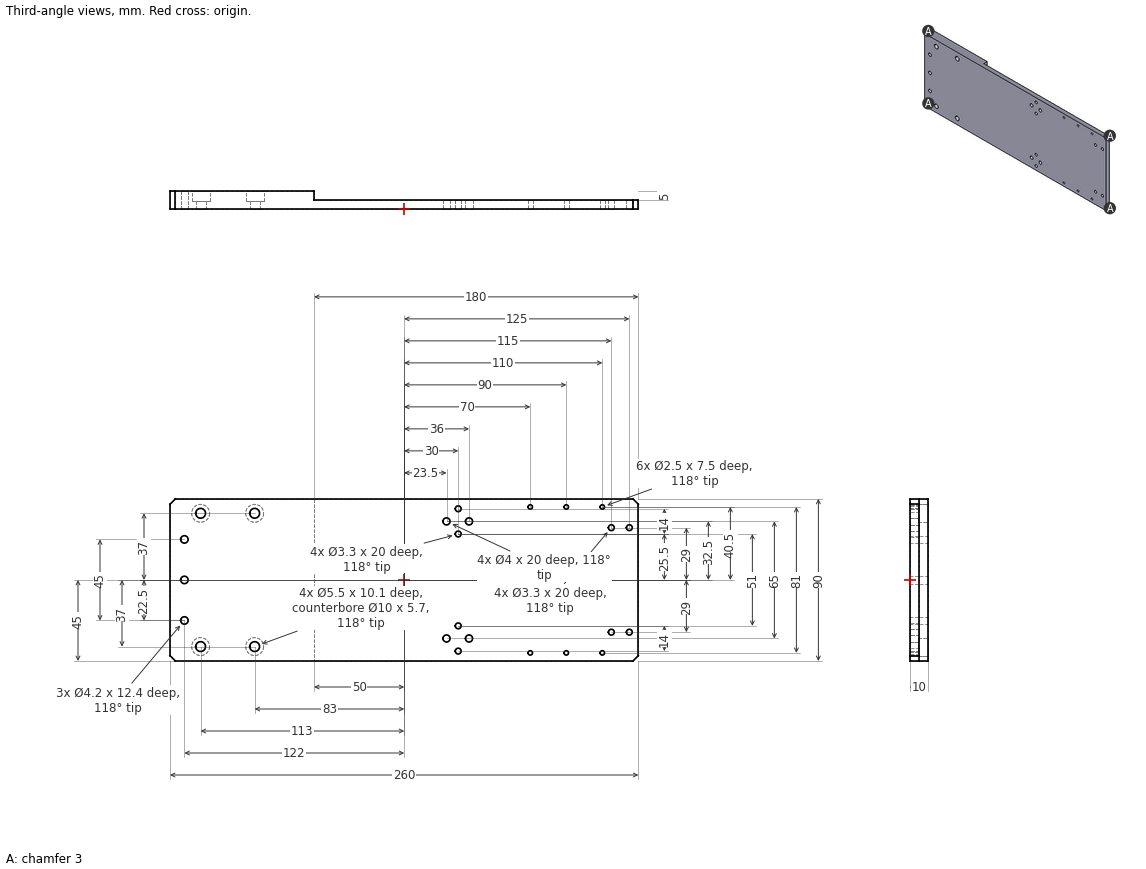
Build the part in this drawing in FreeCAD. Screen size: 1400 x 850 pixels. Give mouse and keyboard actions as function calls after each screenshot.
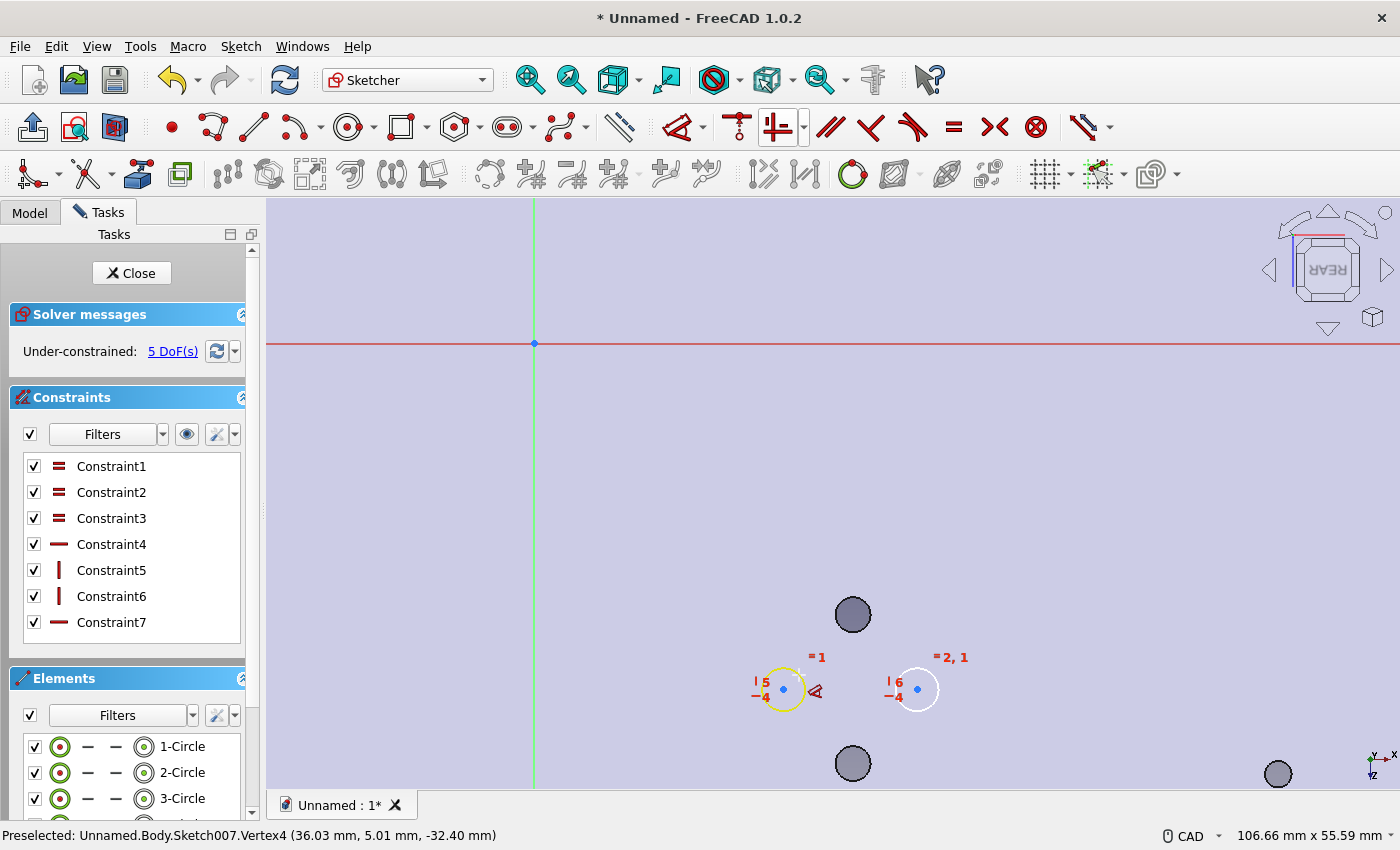
click(799, 675)
click(822, 653)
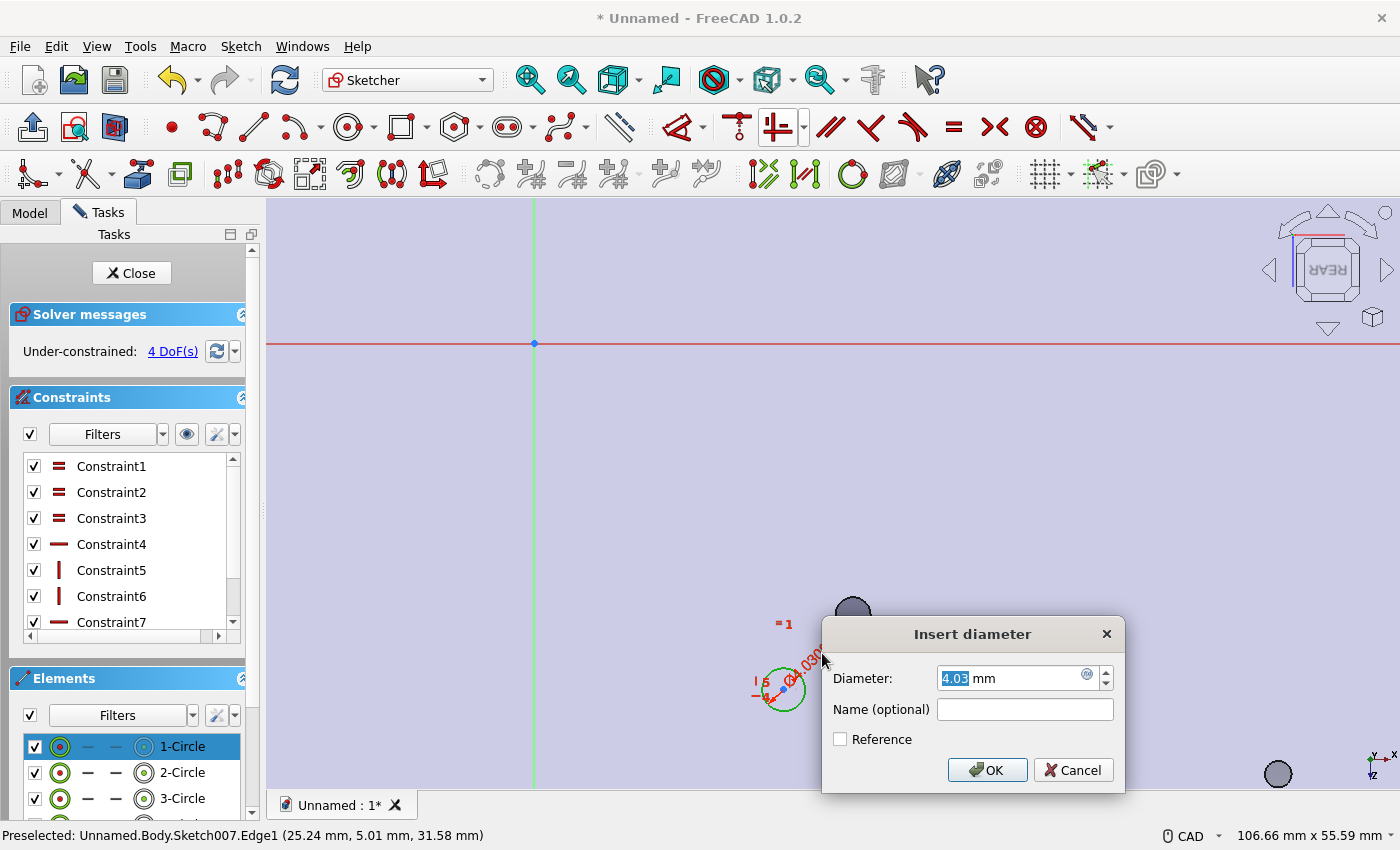
text(4)
key(Return)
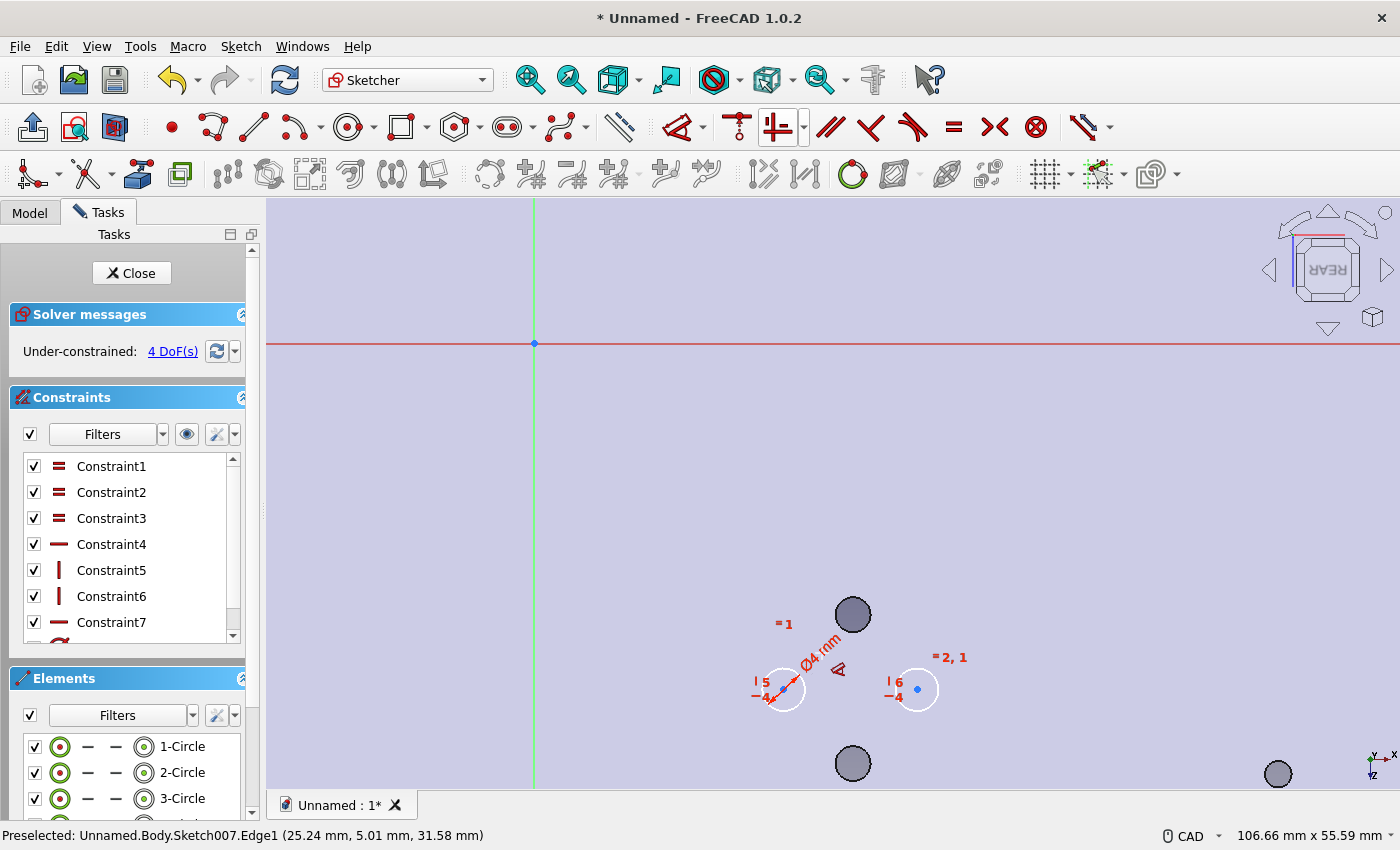
click(917, 690)
click(726, 724)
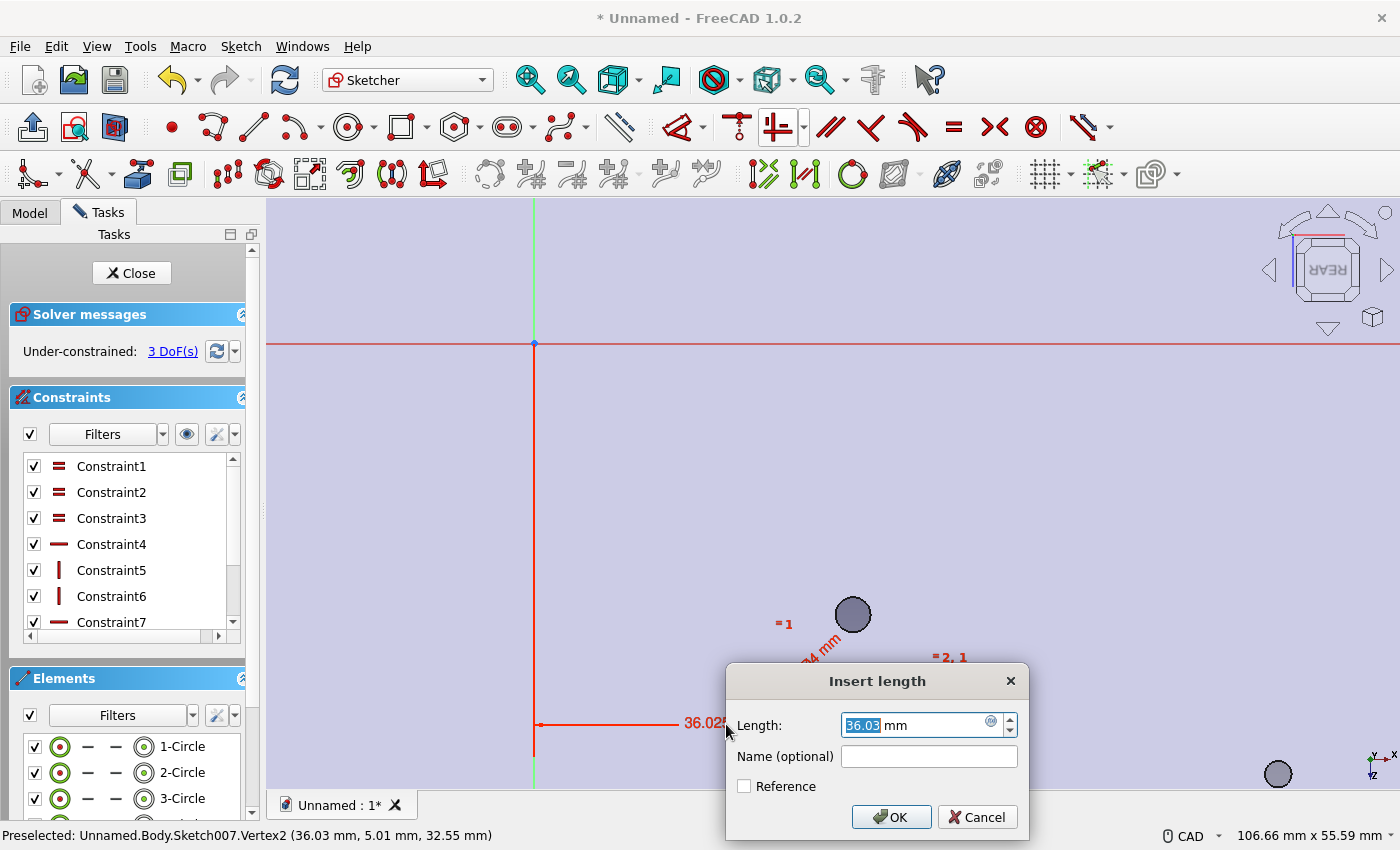
text(36)
key(Return)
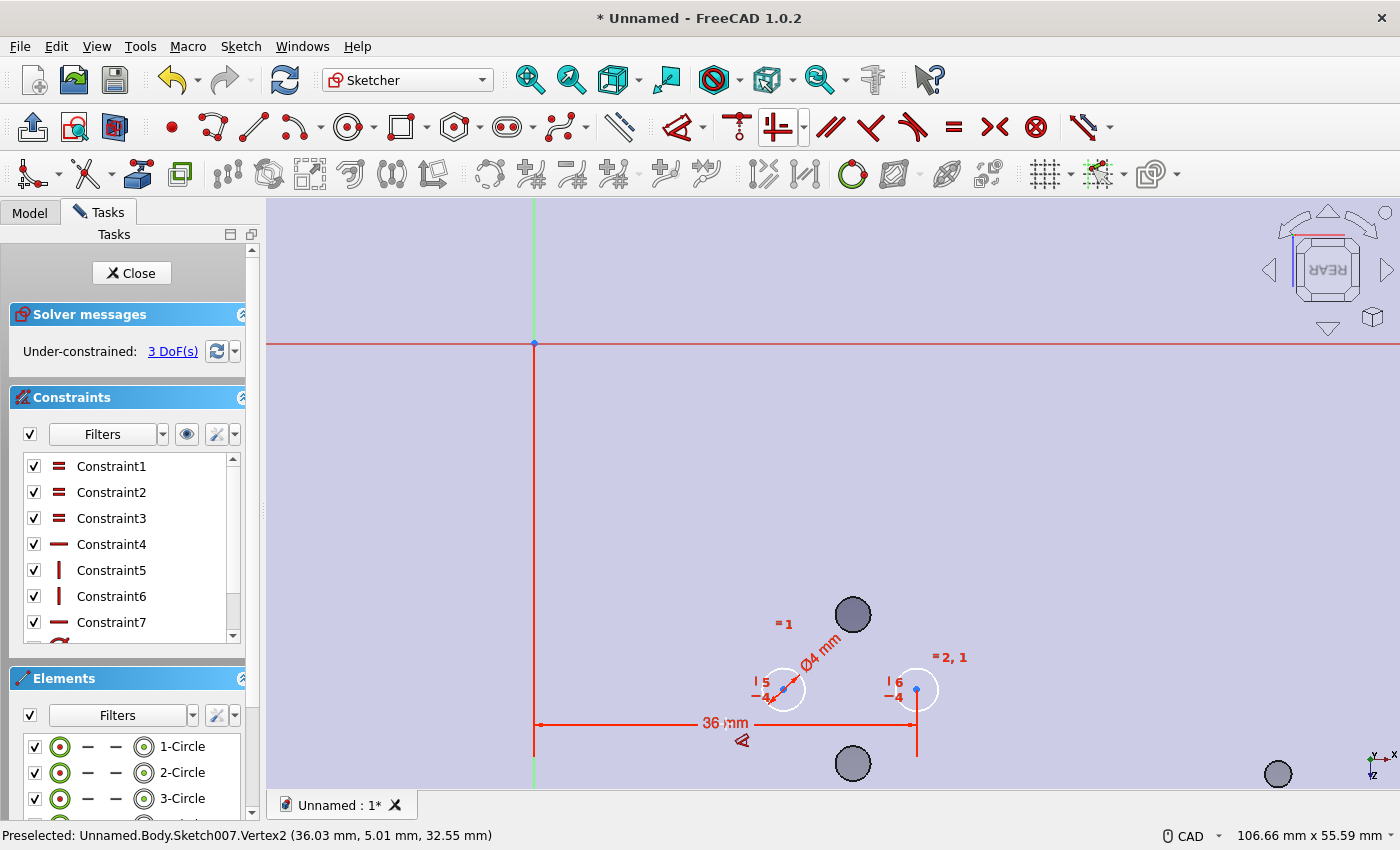
click(784, 690)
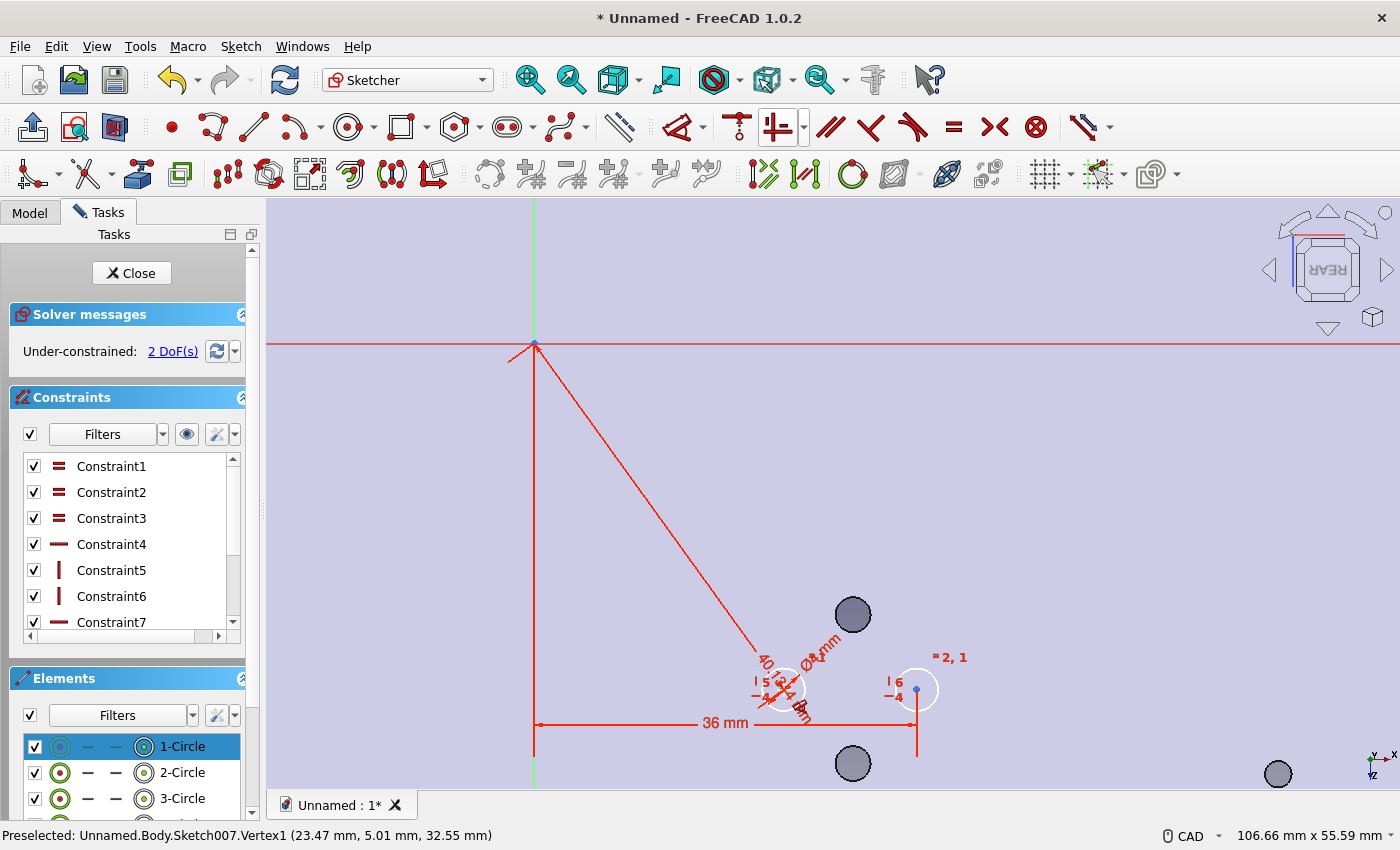
scroll(799, 676, down, 3)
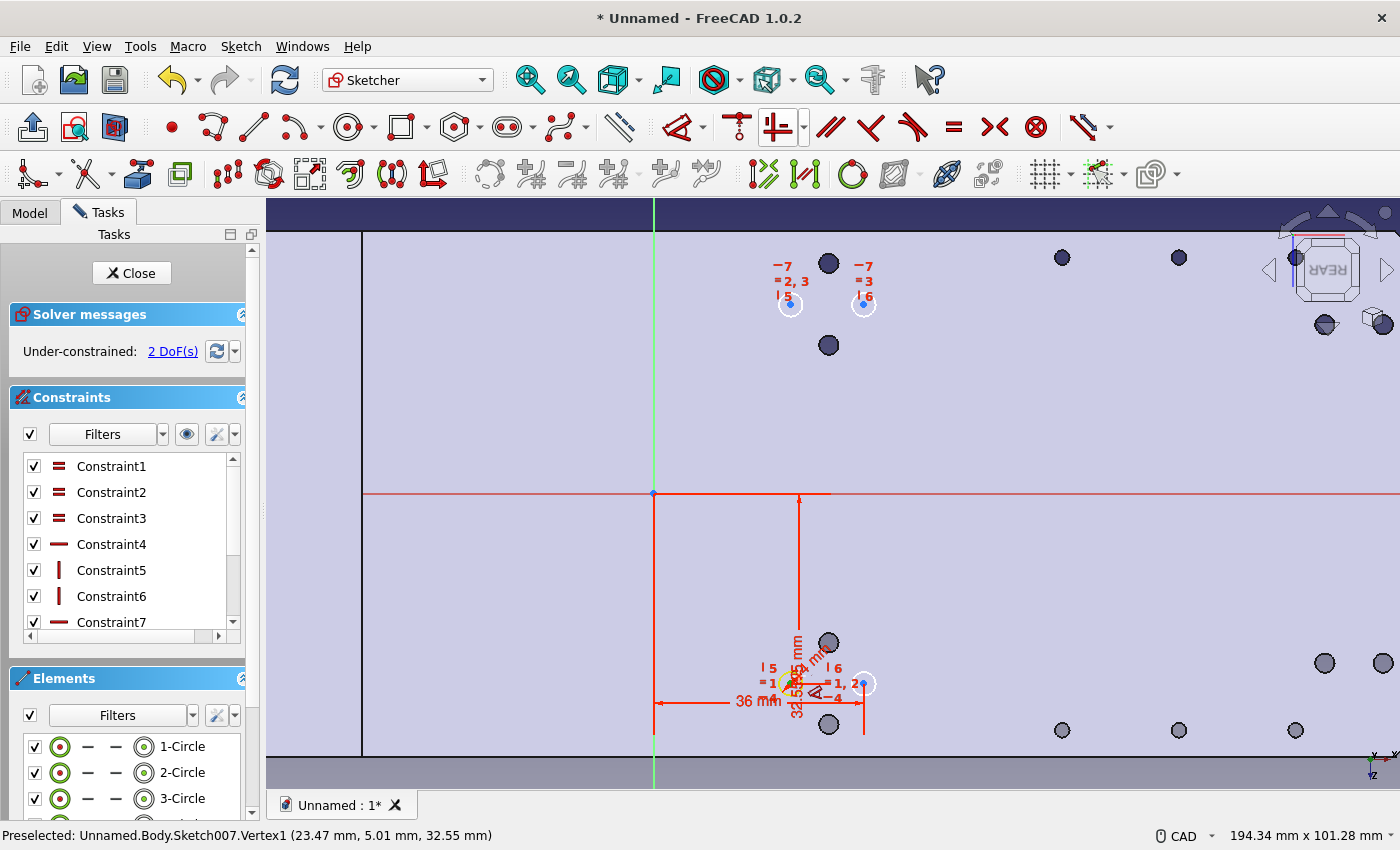
click(791, 305)
click(825, 407)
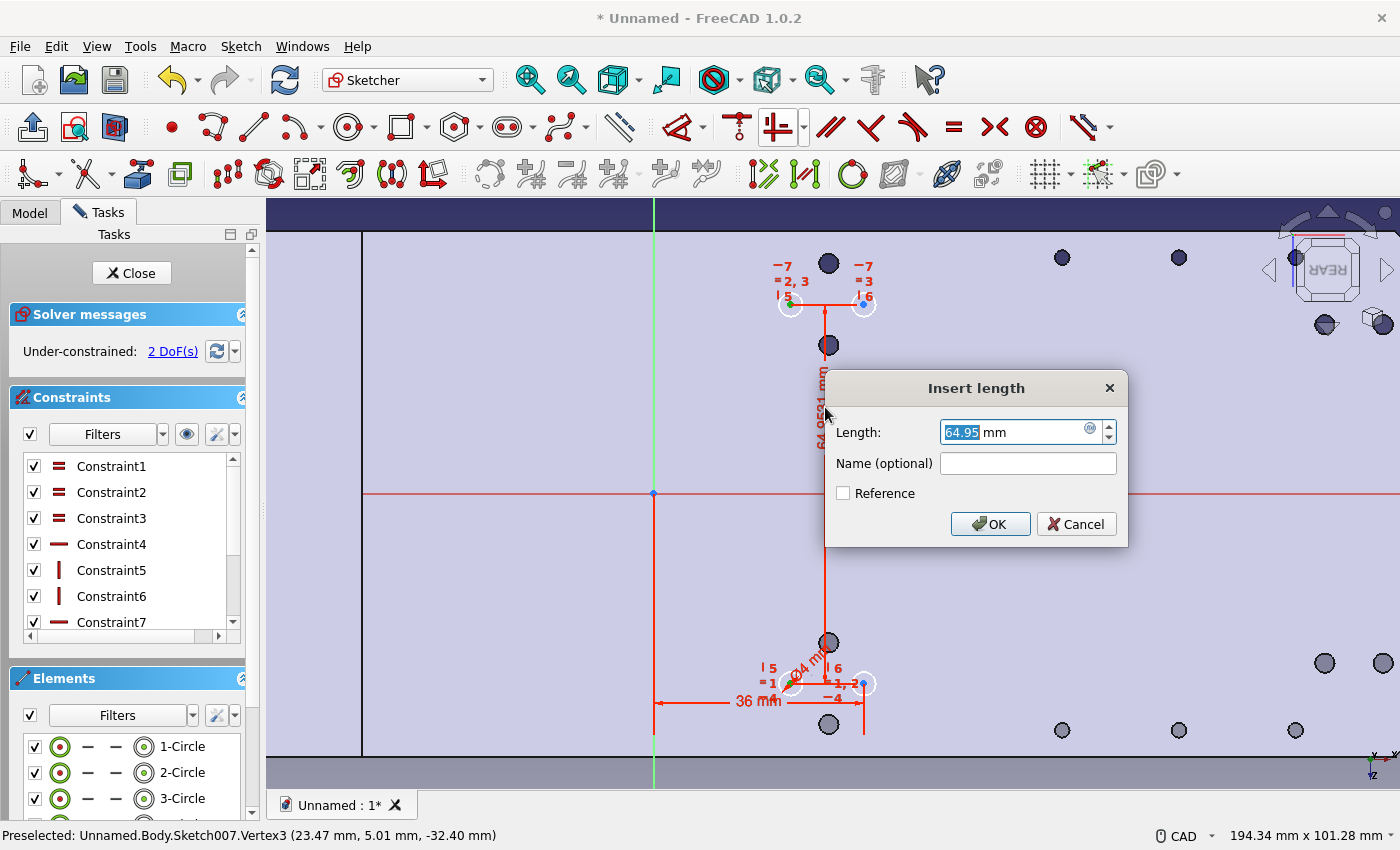
text(65)
key(Return)